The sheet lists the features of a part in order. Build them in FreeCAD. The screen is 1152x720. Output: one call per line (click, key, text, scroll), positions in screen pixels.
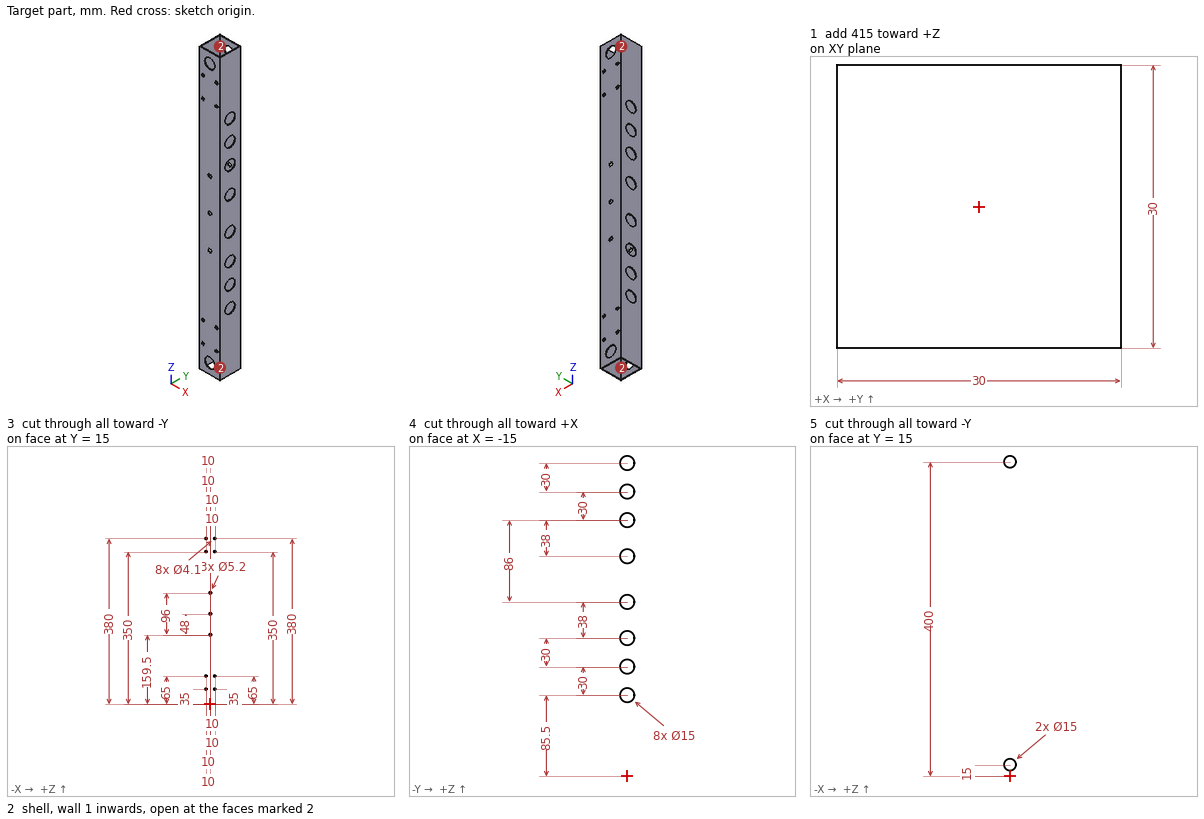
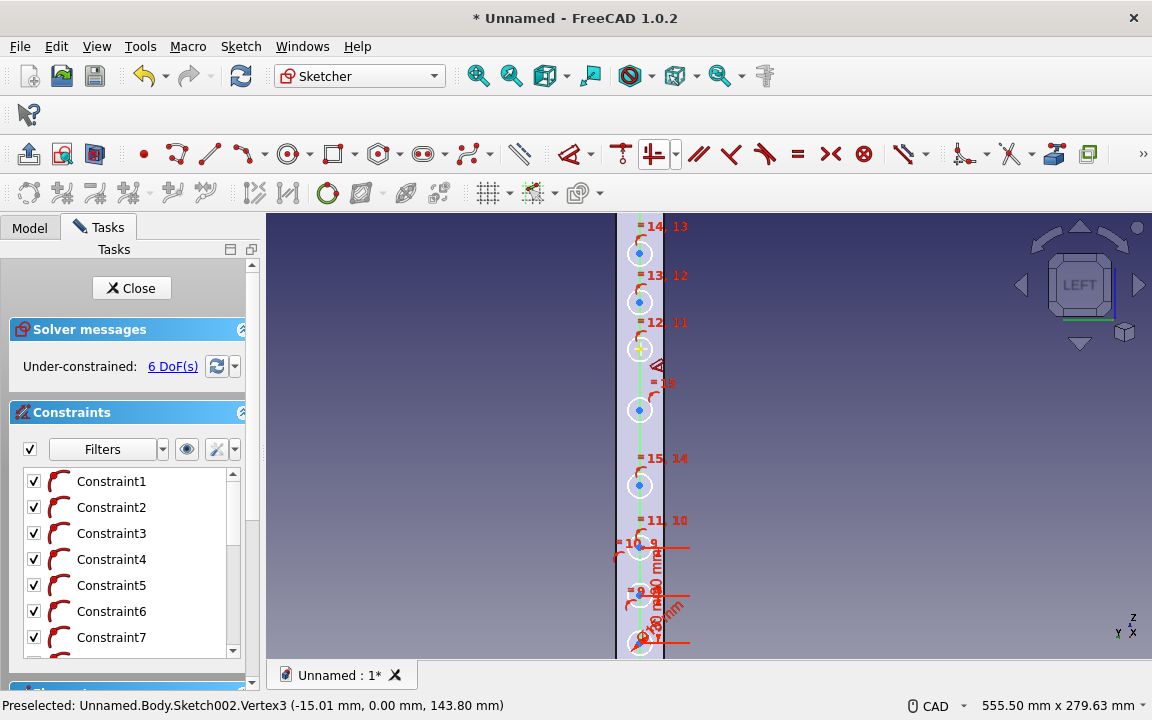
click(640, 350)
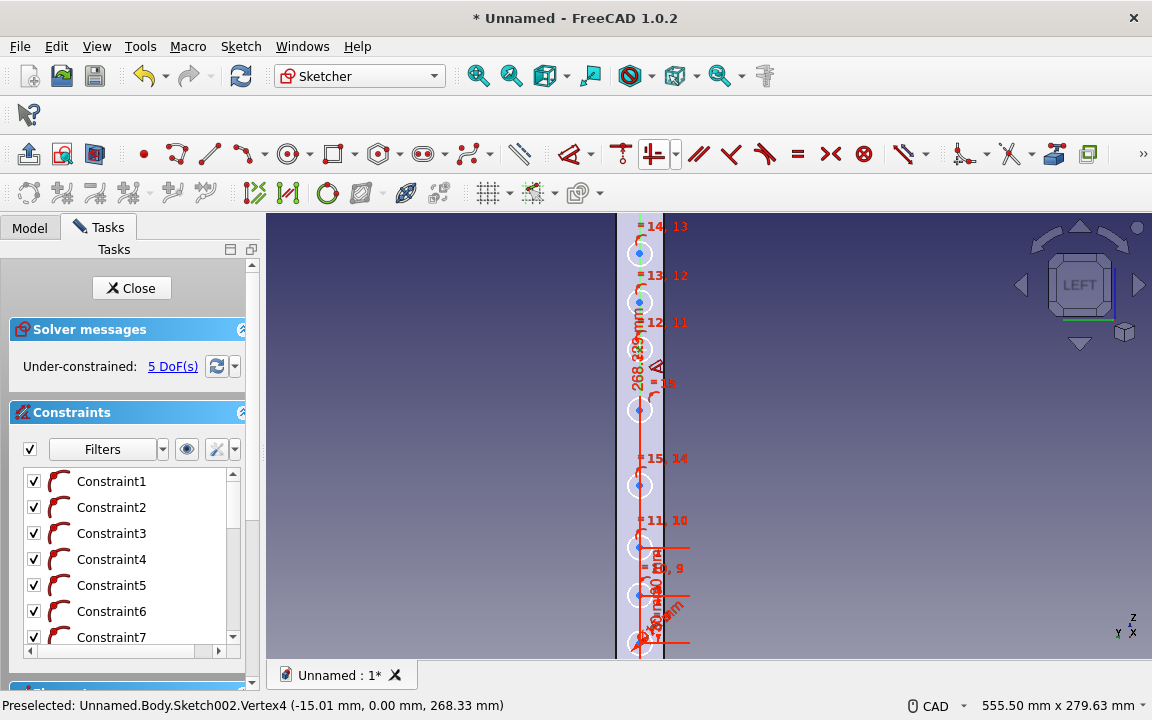
click(640, 302)
click(674, 326)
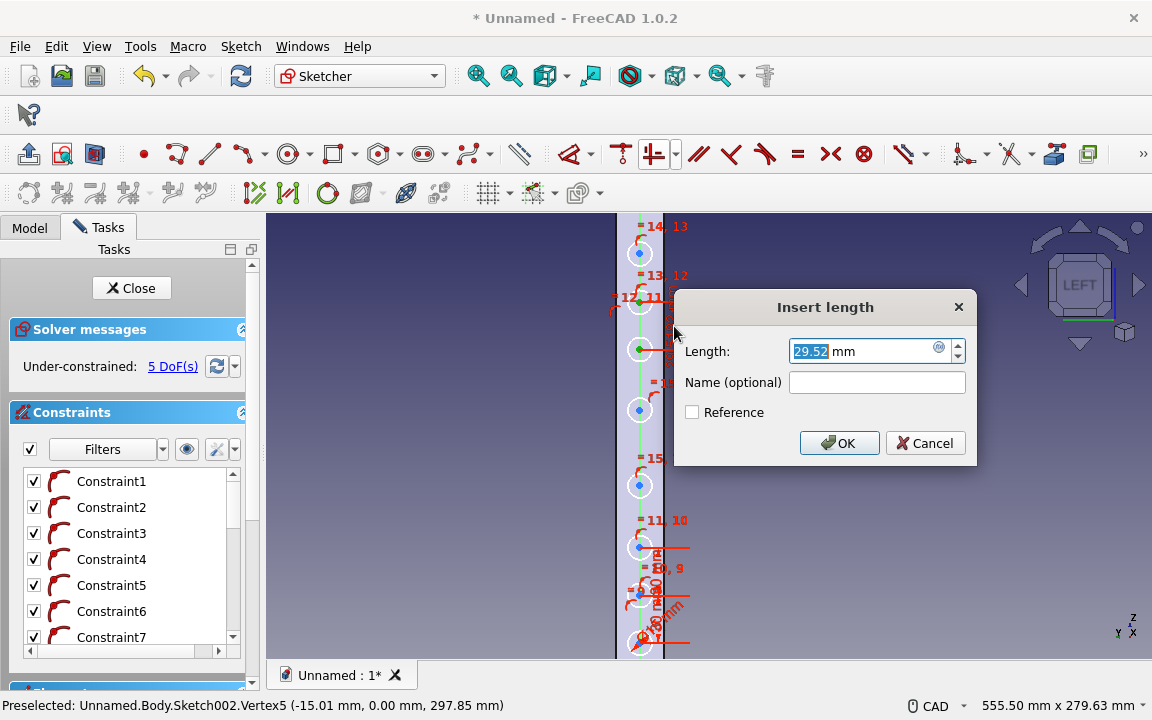
text(30)
key(Return)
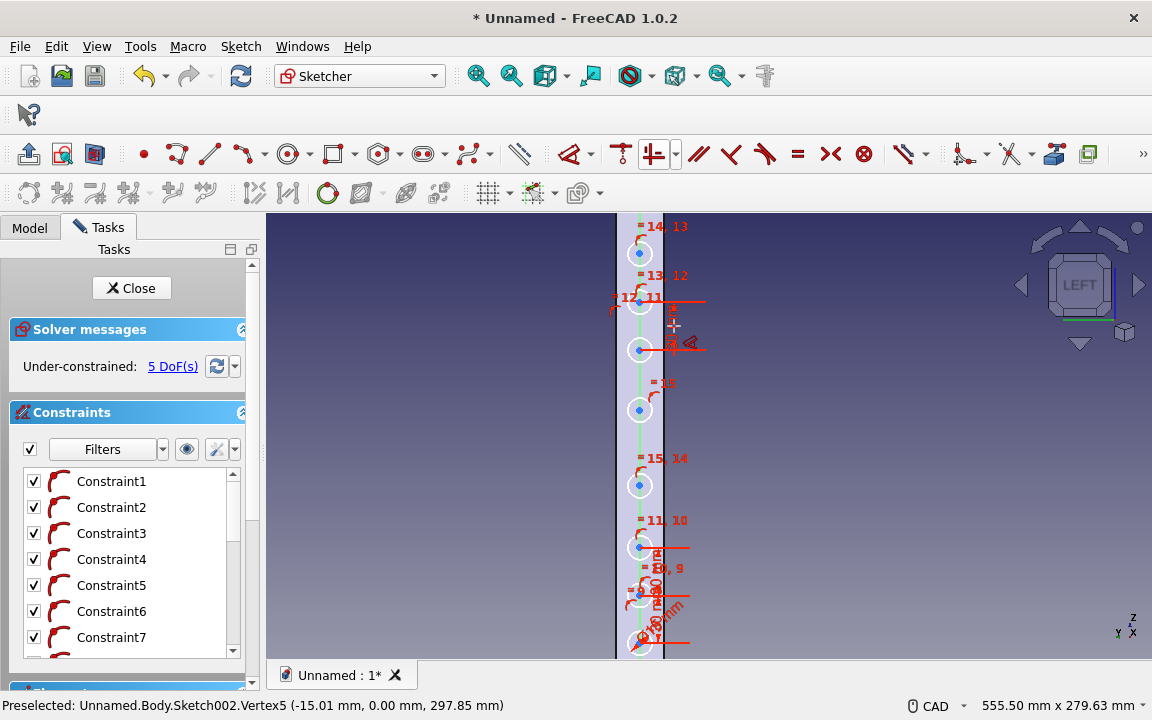
click(640, 302)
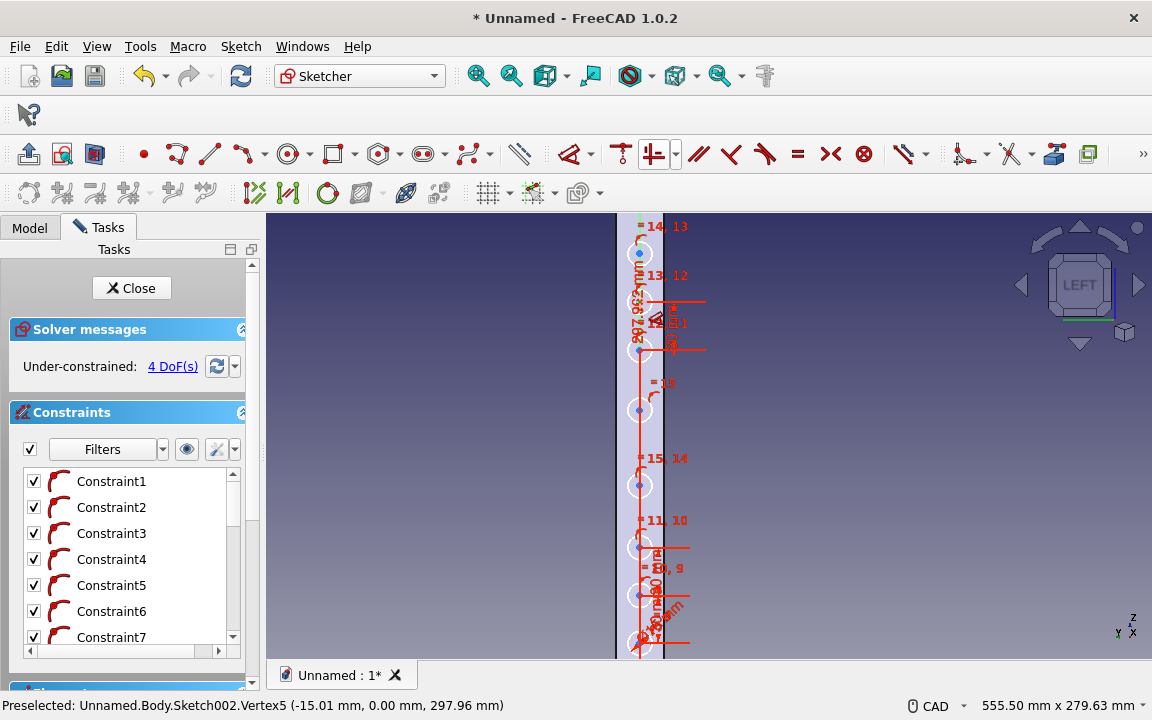
click(640, 254)
click(674, 278)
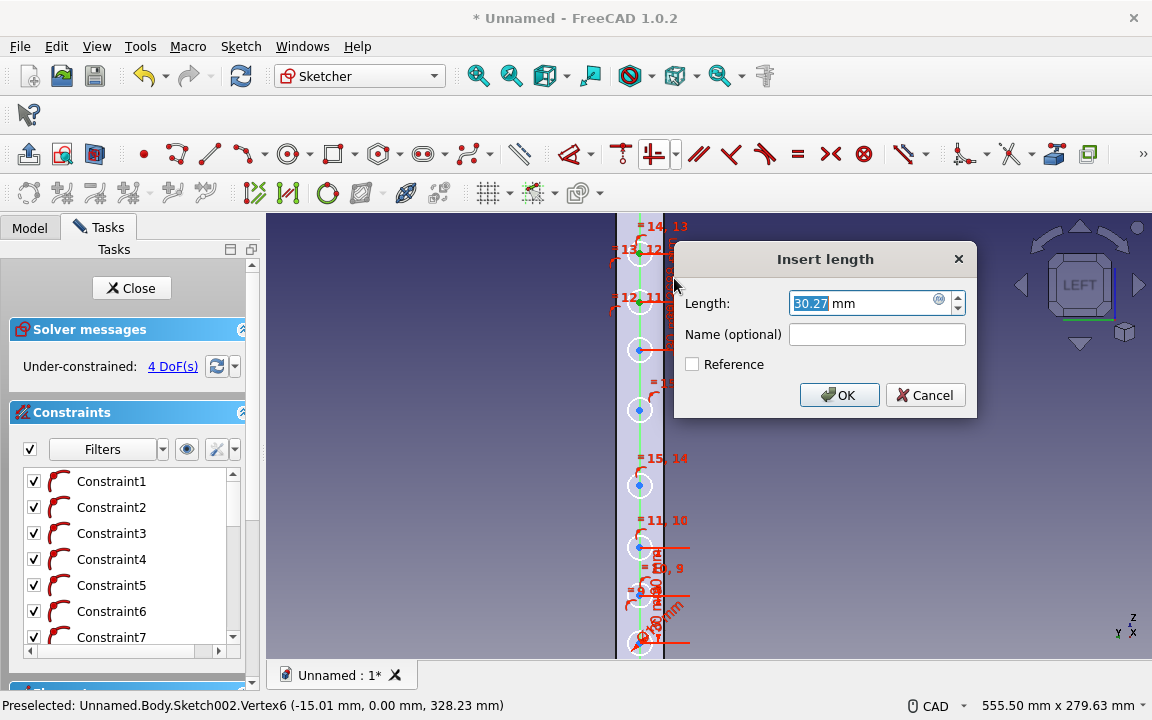
text(30)
key(Return)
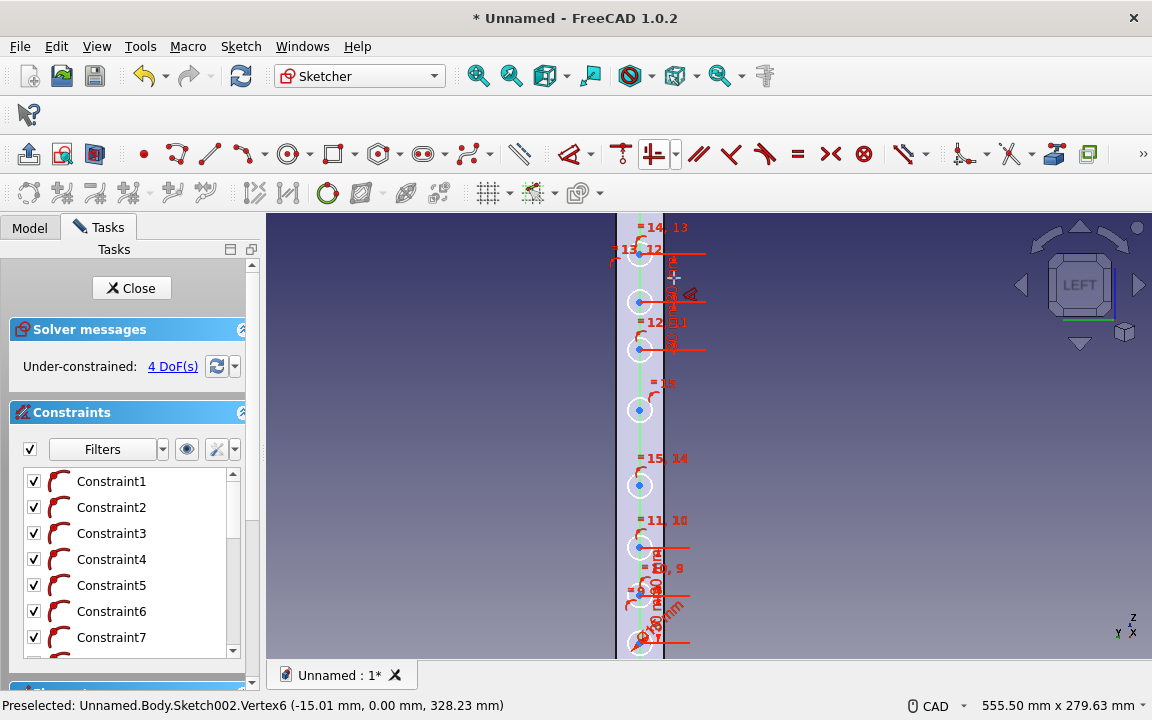
click(640, 548)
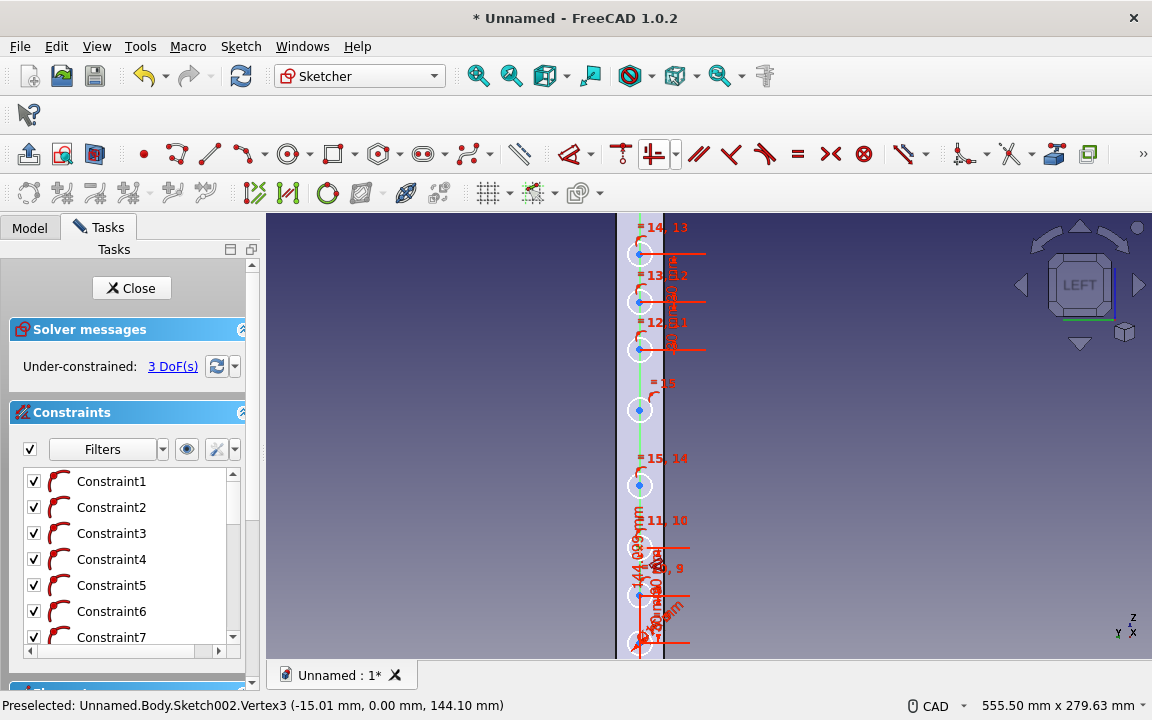
click(640, 486)
click(674, 517)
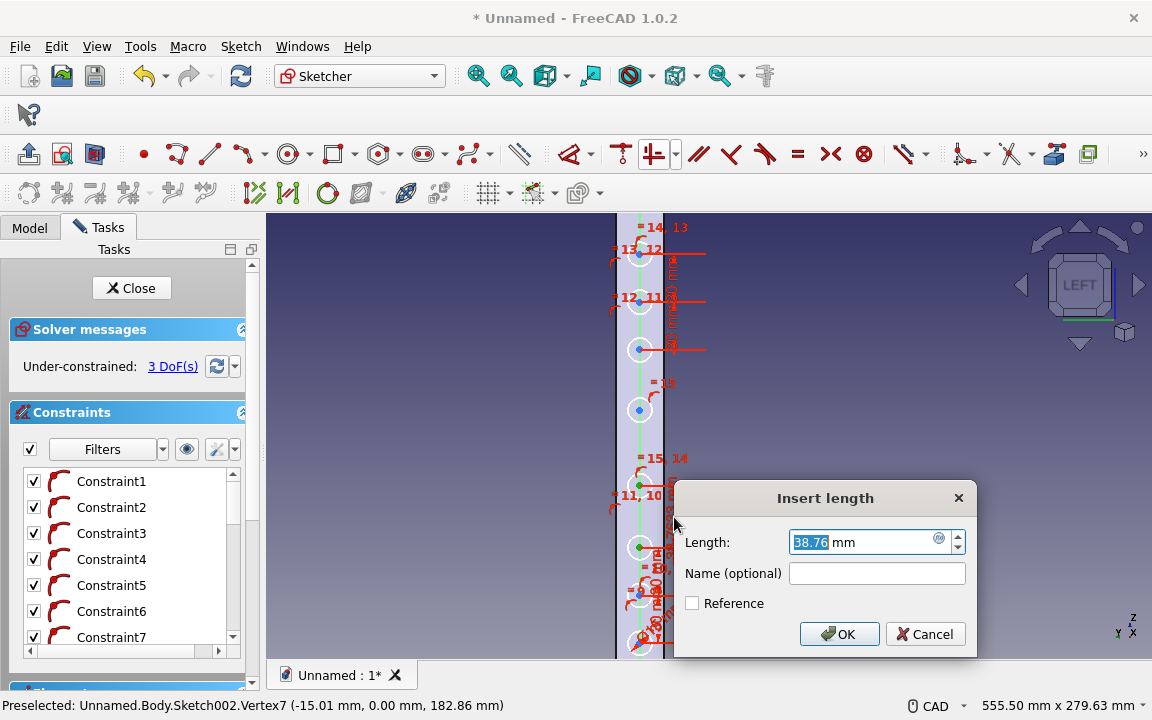
text(38)
key(Return)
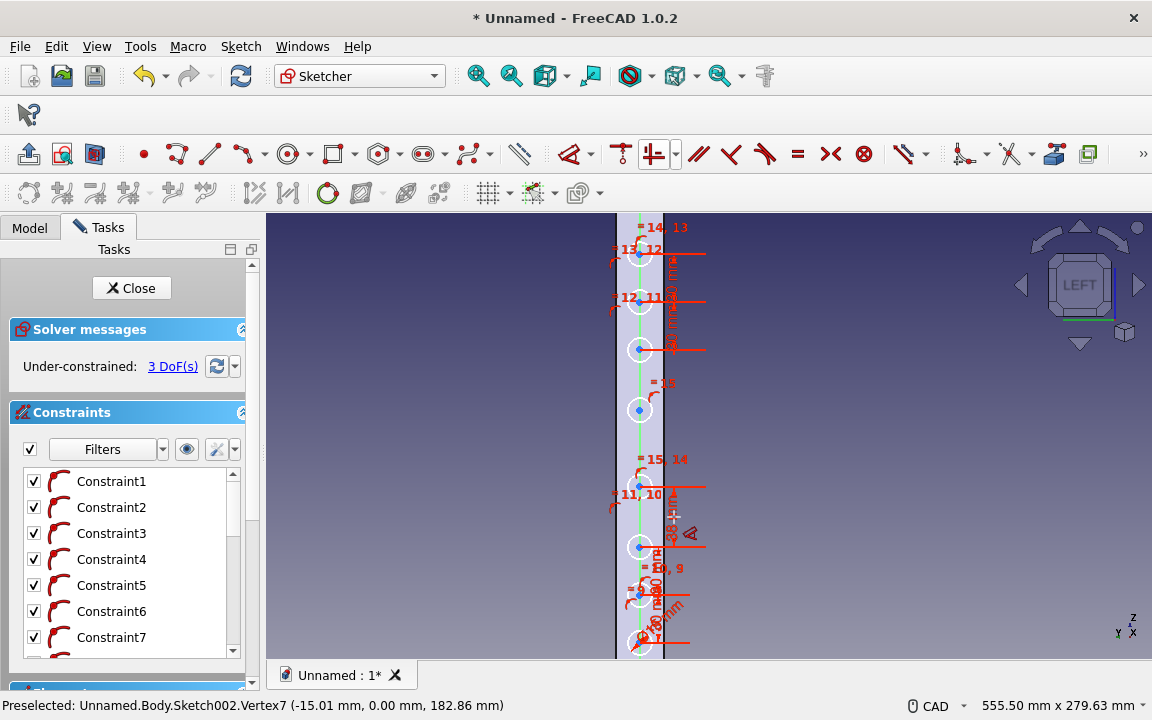
click(640, 350)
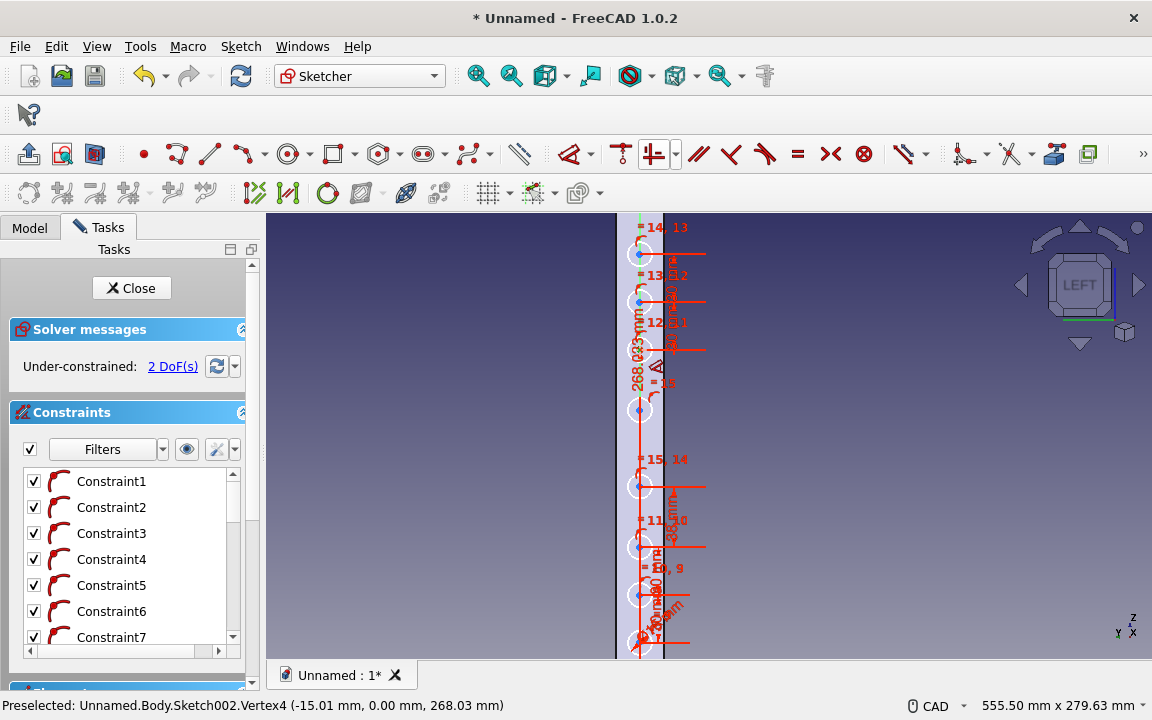
click(640, 487)
click(674, 418)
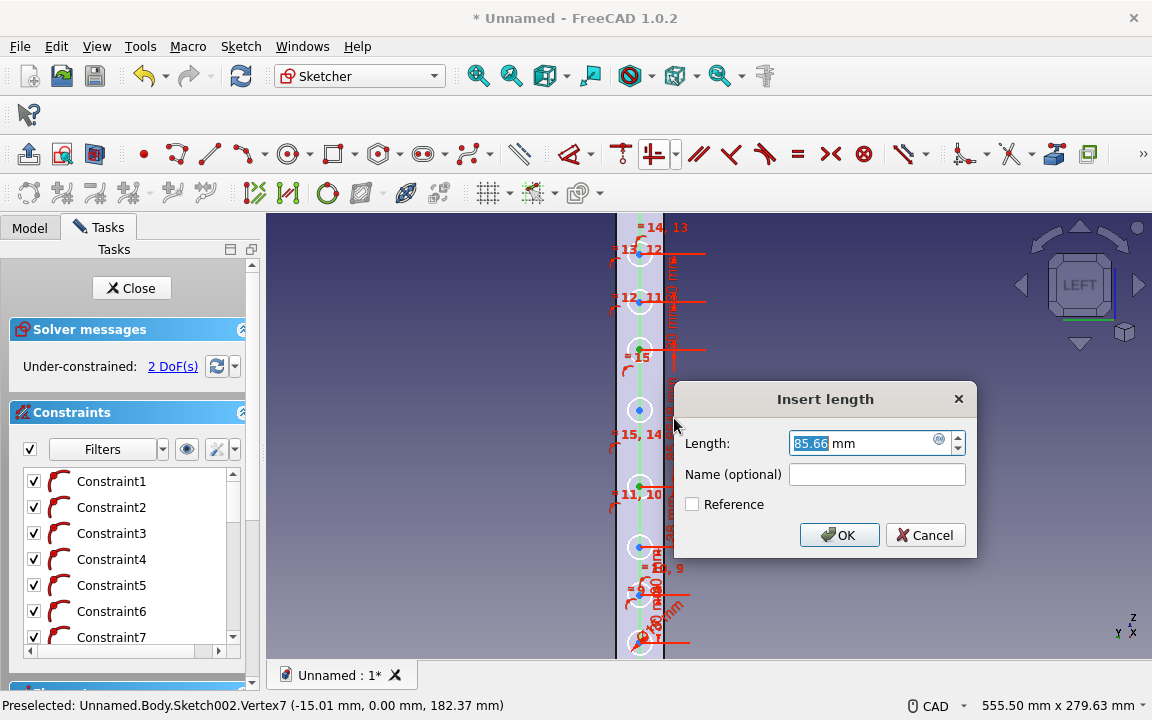
text(86)
key(Return)